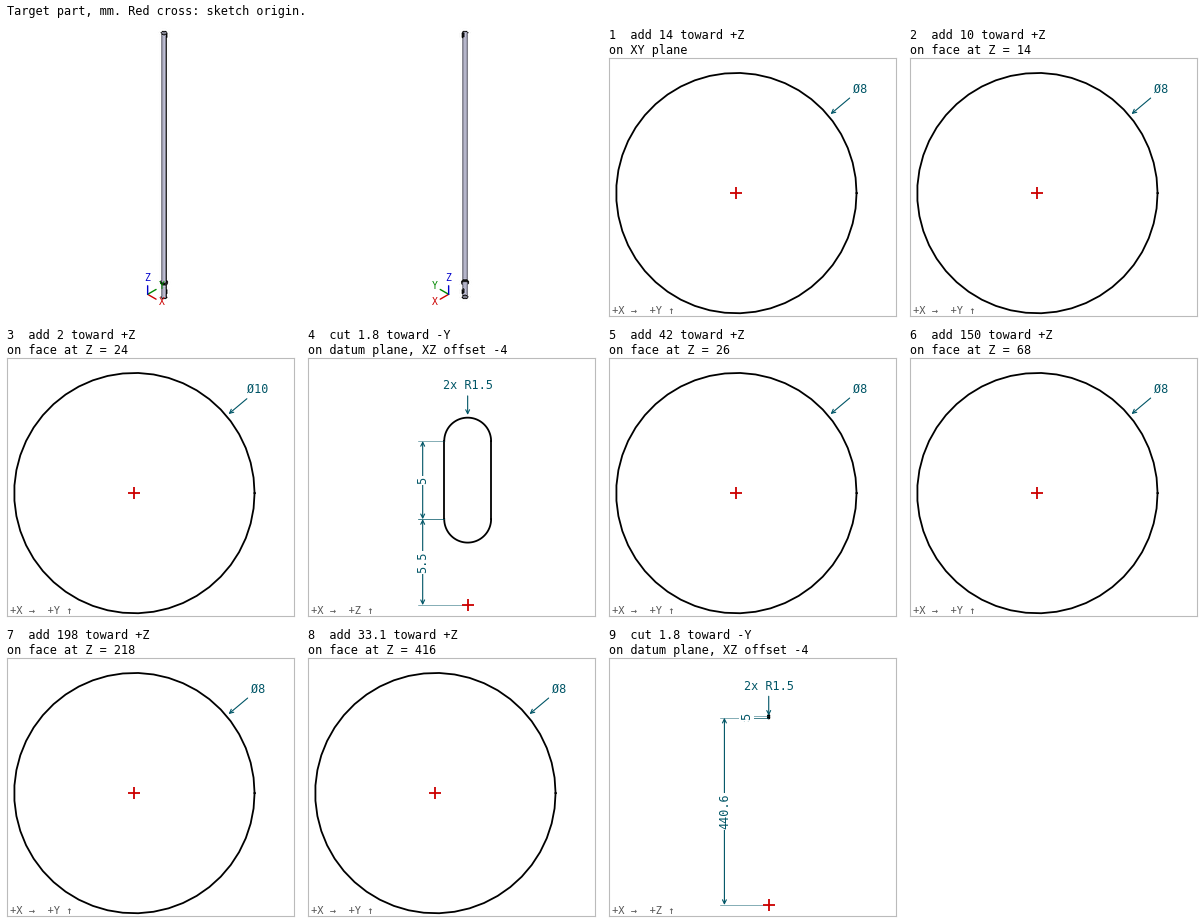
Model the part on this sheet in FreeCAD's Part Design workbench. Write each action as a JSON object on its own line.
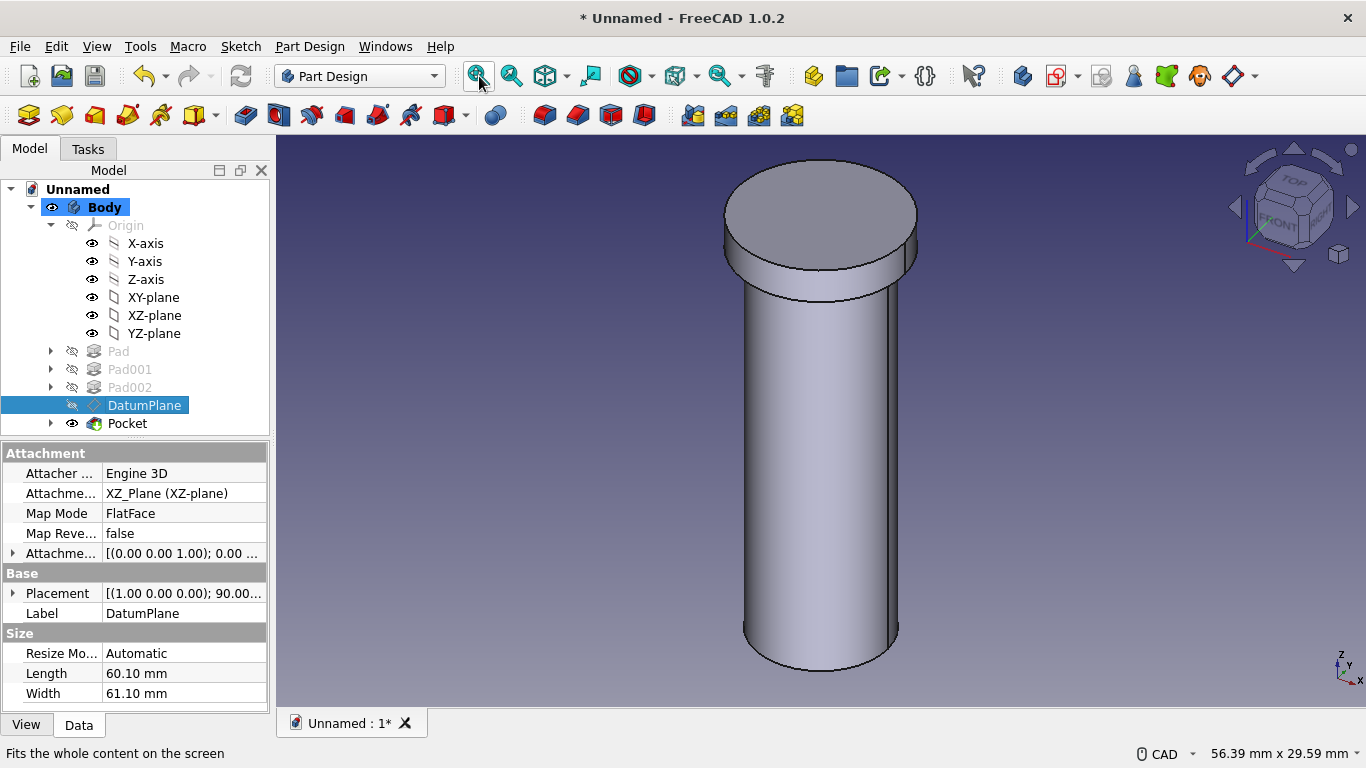
{"action": "left_click", "coordinate": [821, 214]}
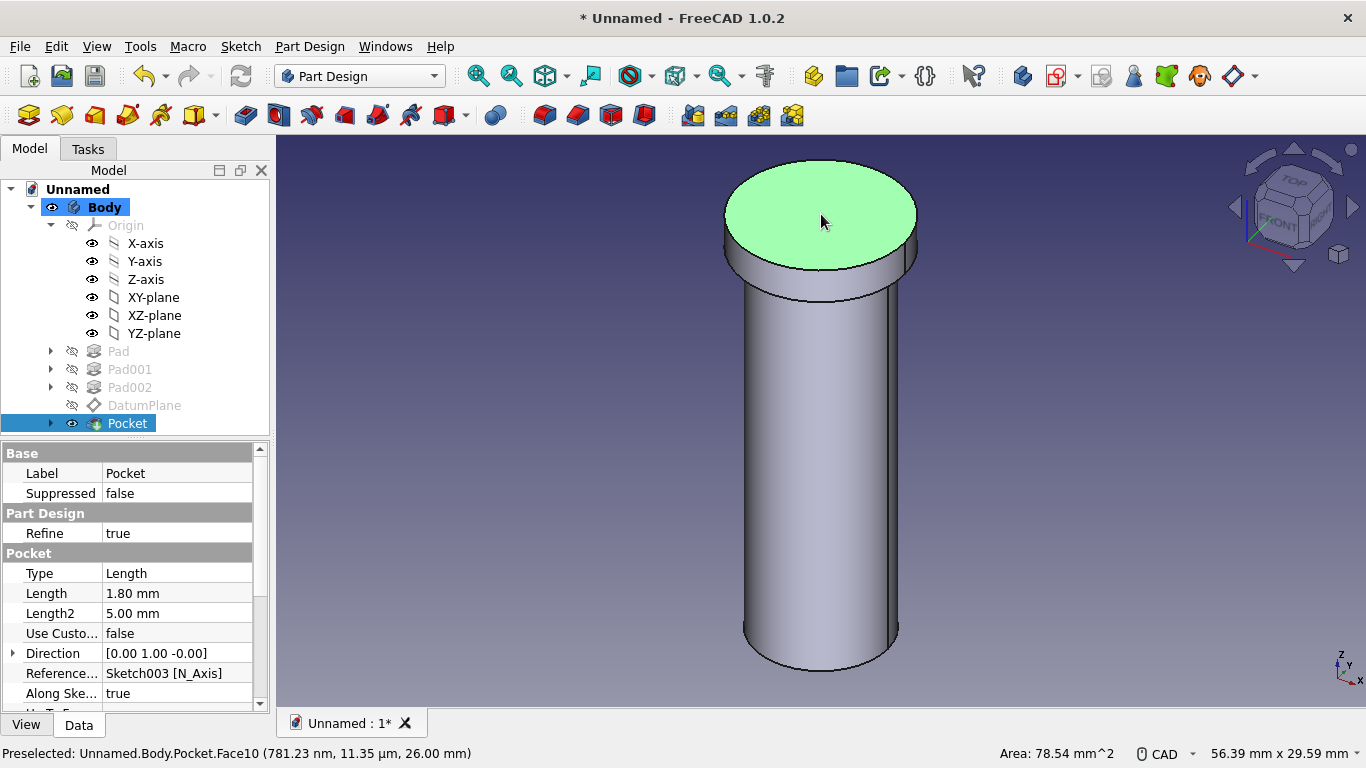
{"action": "left_click", "coordinate": [1056, 76]}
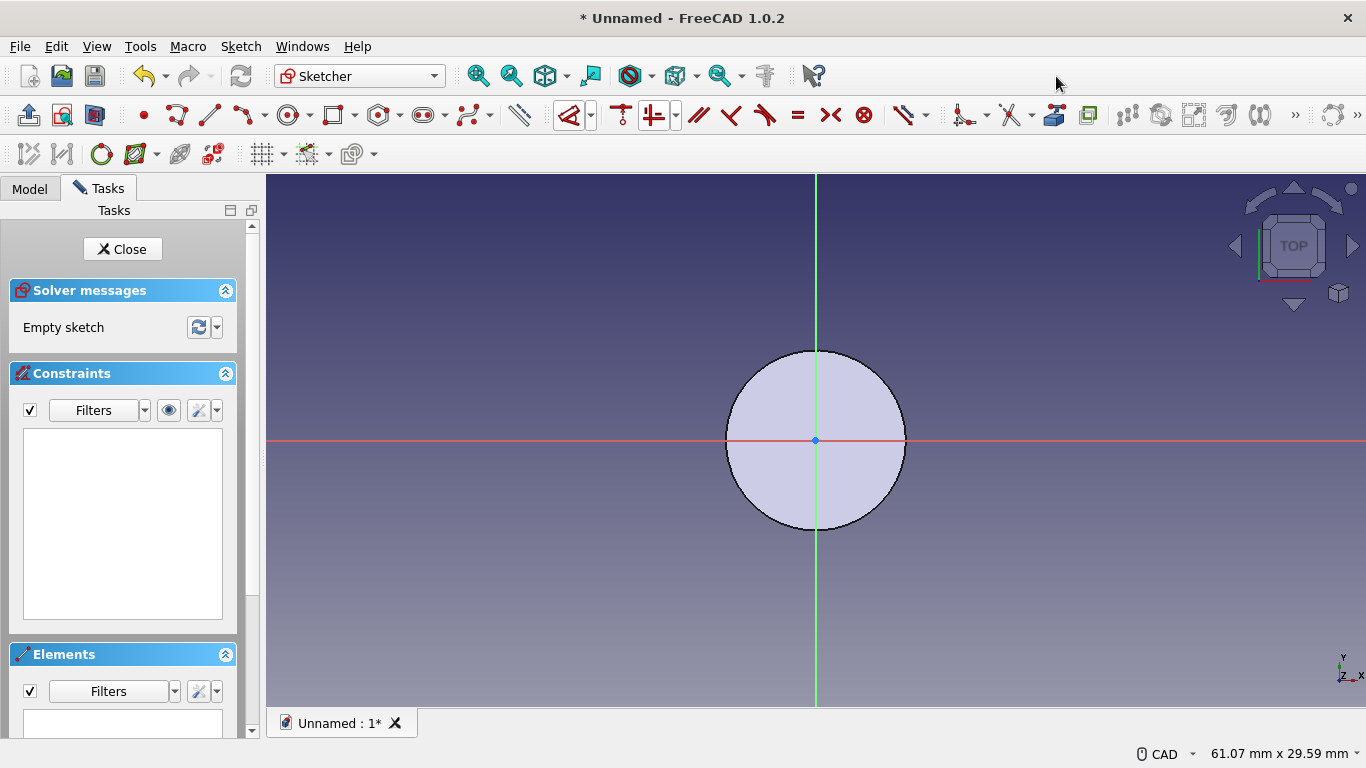
{"action": "scroll", "coordinate": [872, 440], "scroll_direction": "up", "scroll_amount": 4}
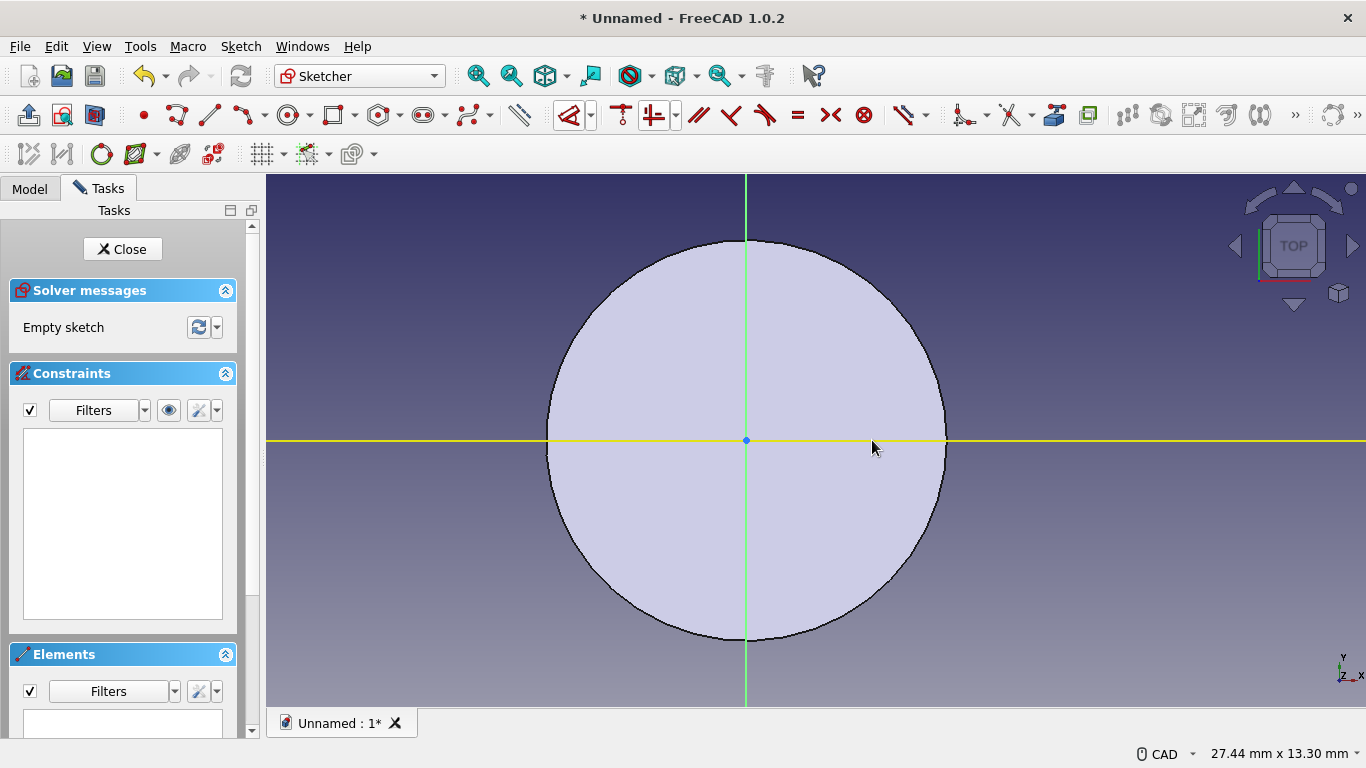
{"action": "left_click", "coordinate": [288, 116]}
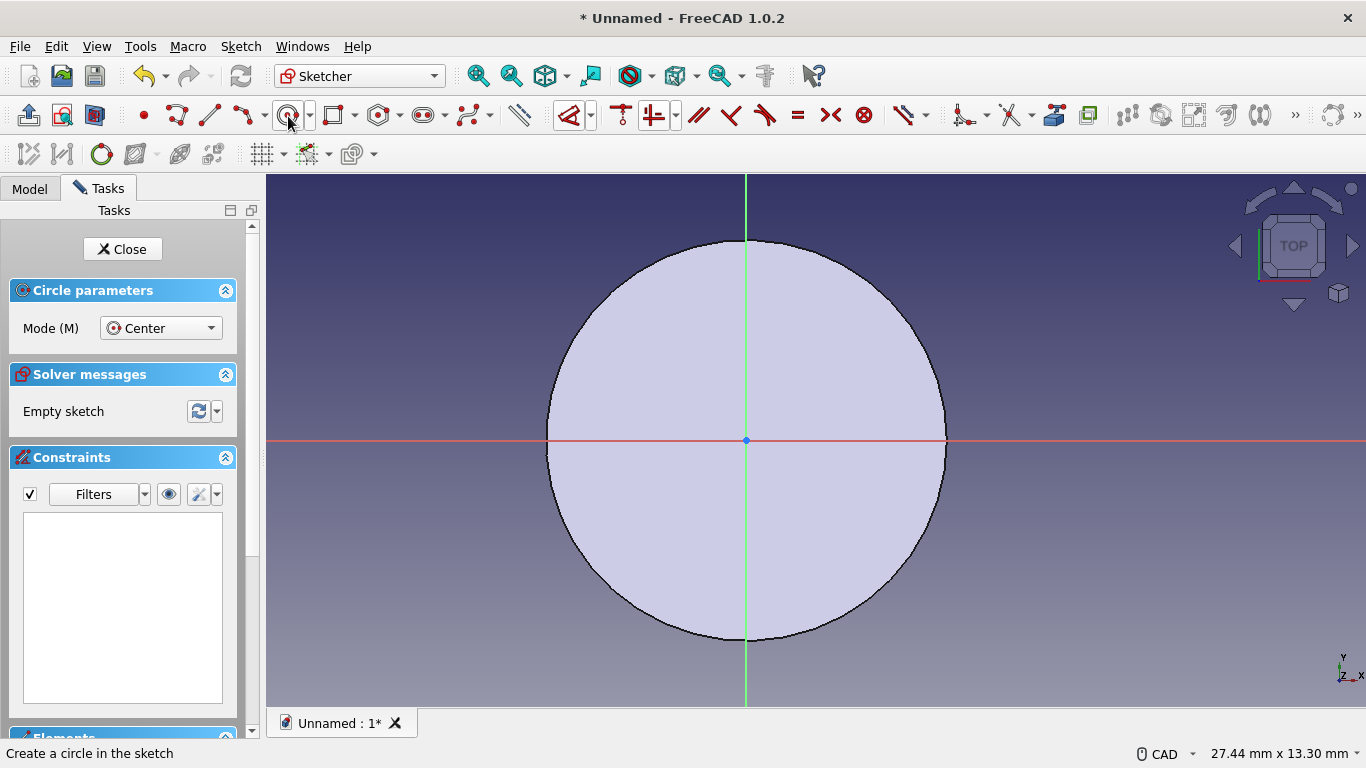
{"action": "left_click", "coordinate": [746, 440]}
{"action": "left_click", "coordinate": [860, 327]}
{"action": "key", "text": "Escape"}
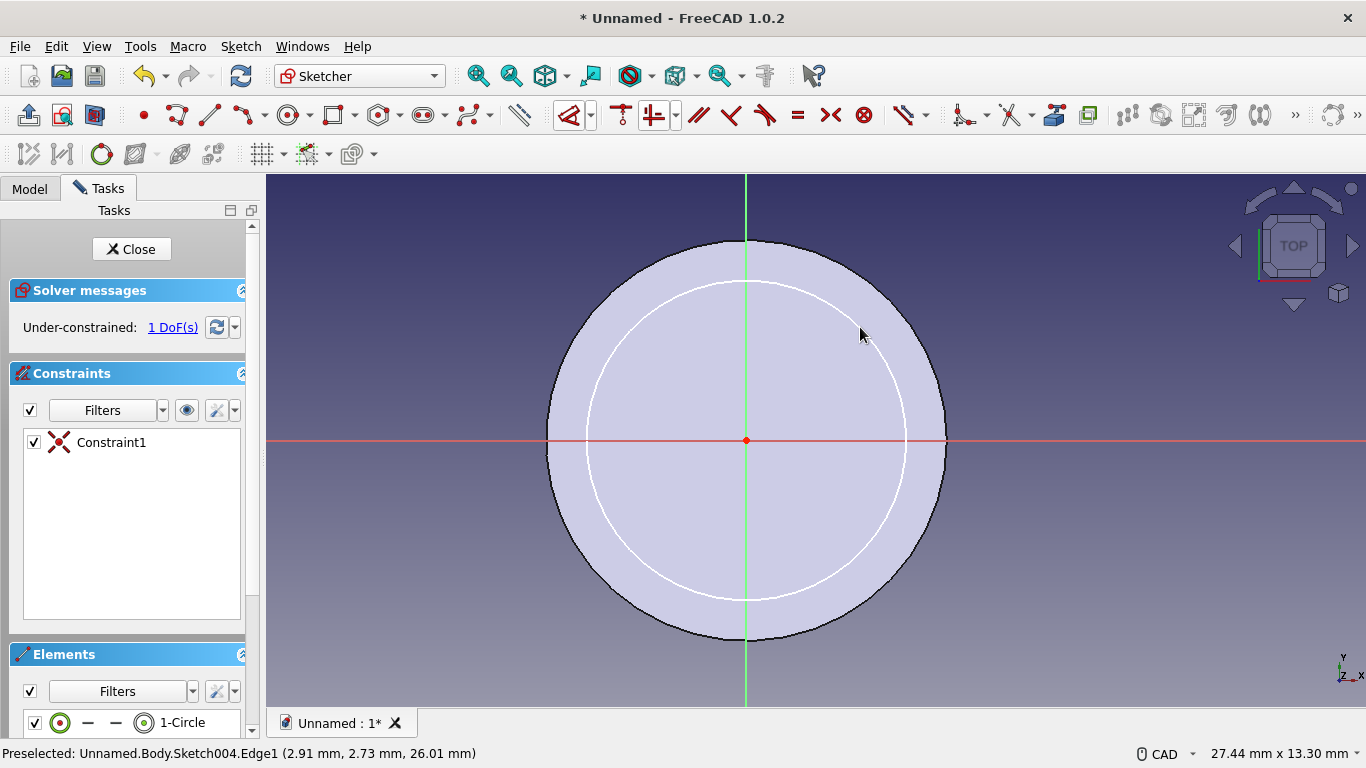
{"action": "left_click", "coordinate": [859, 327]}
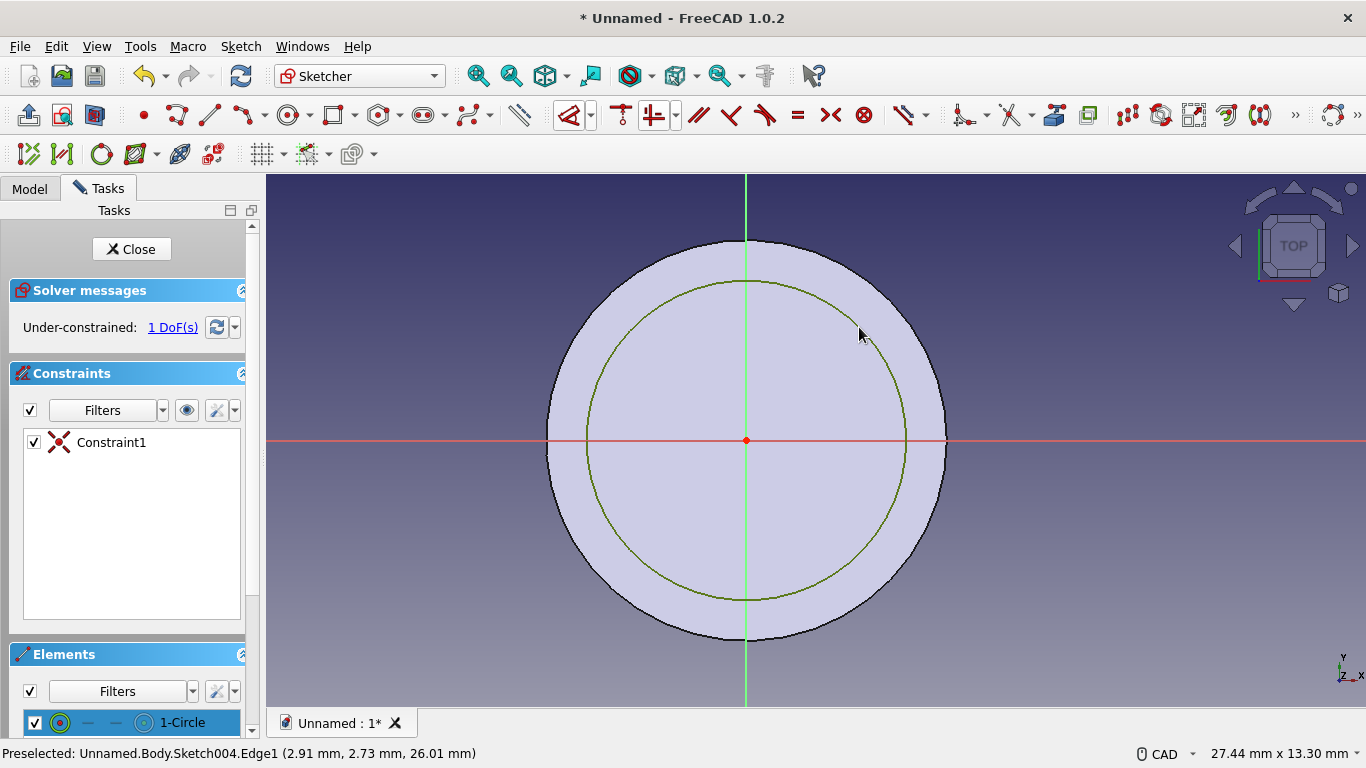
{"action": "key", "text": "k o"}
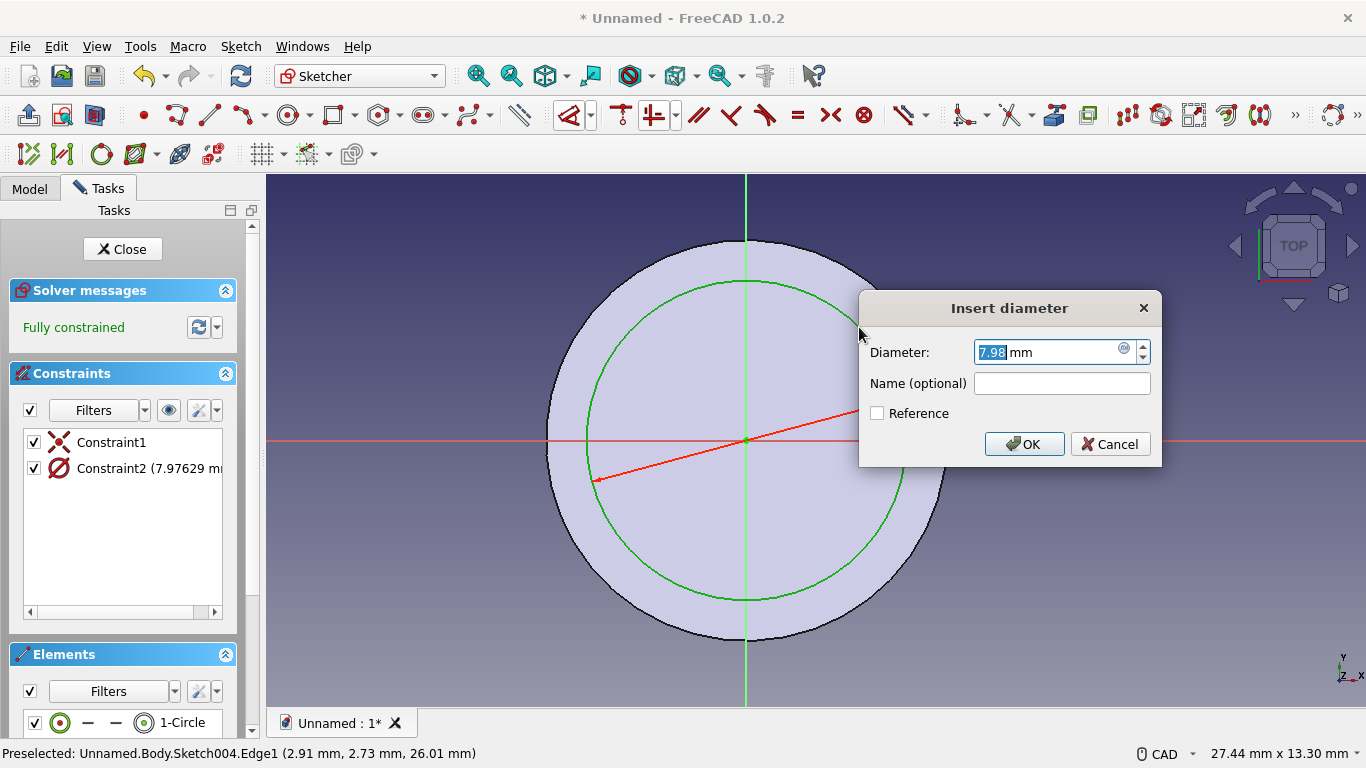
{"action": "type", "text": "8"}
{"action": "key", "text": "Return"}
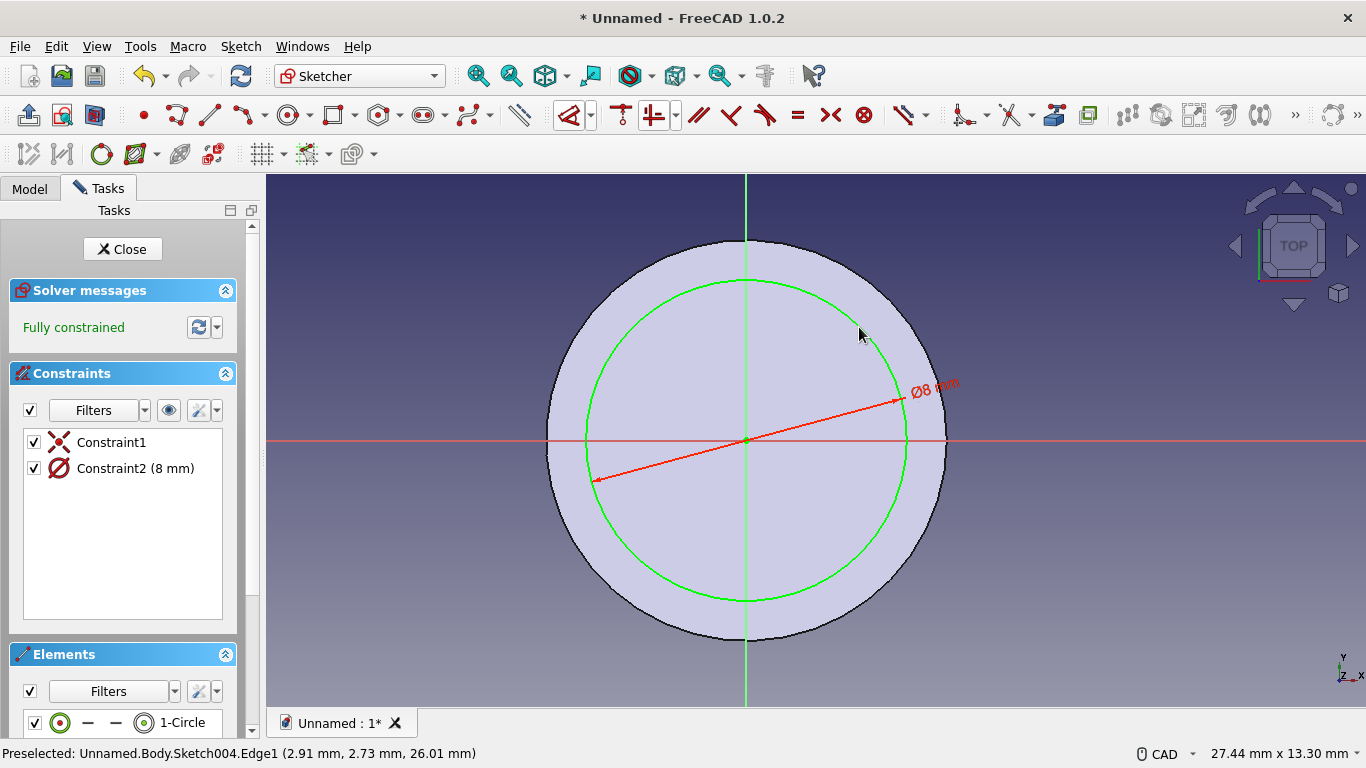
{"action": "left_click", "coordinate": [123, 249]}